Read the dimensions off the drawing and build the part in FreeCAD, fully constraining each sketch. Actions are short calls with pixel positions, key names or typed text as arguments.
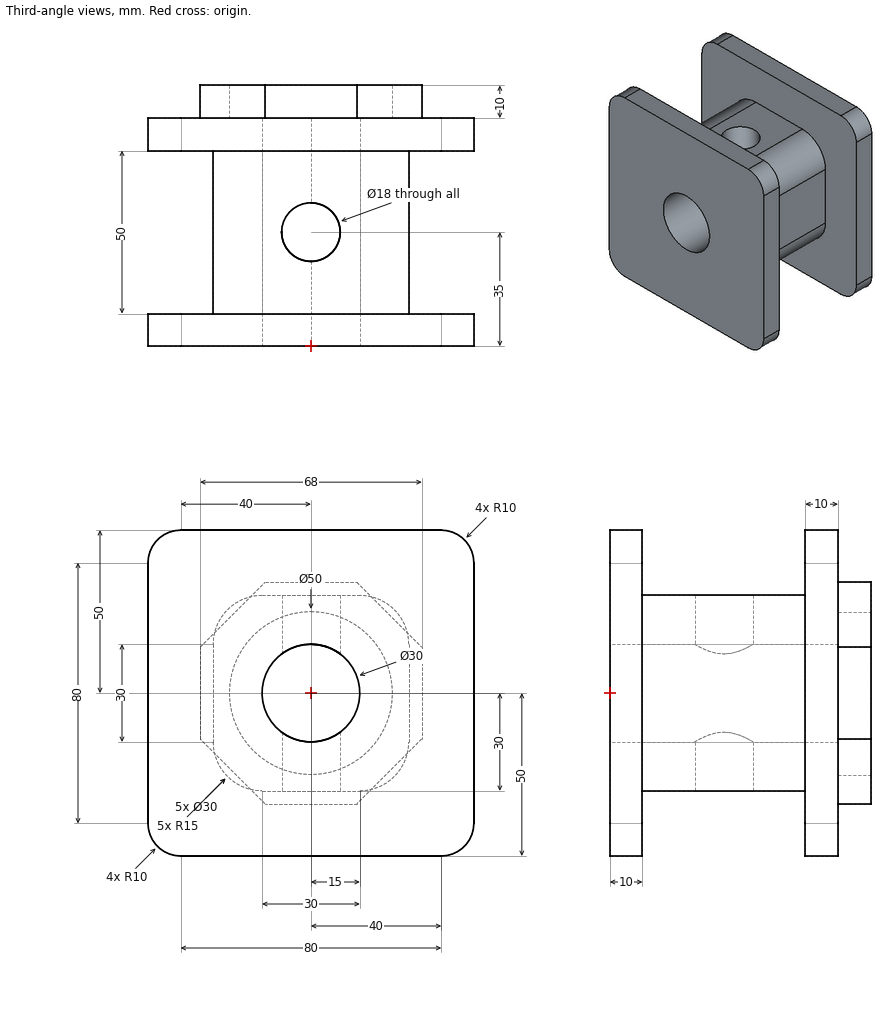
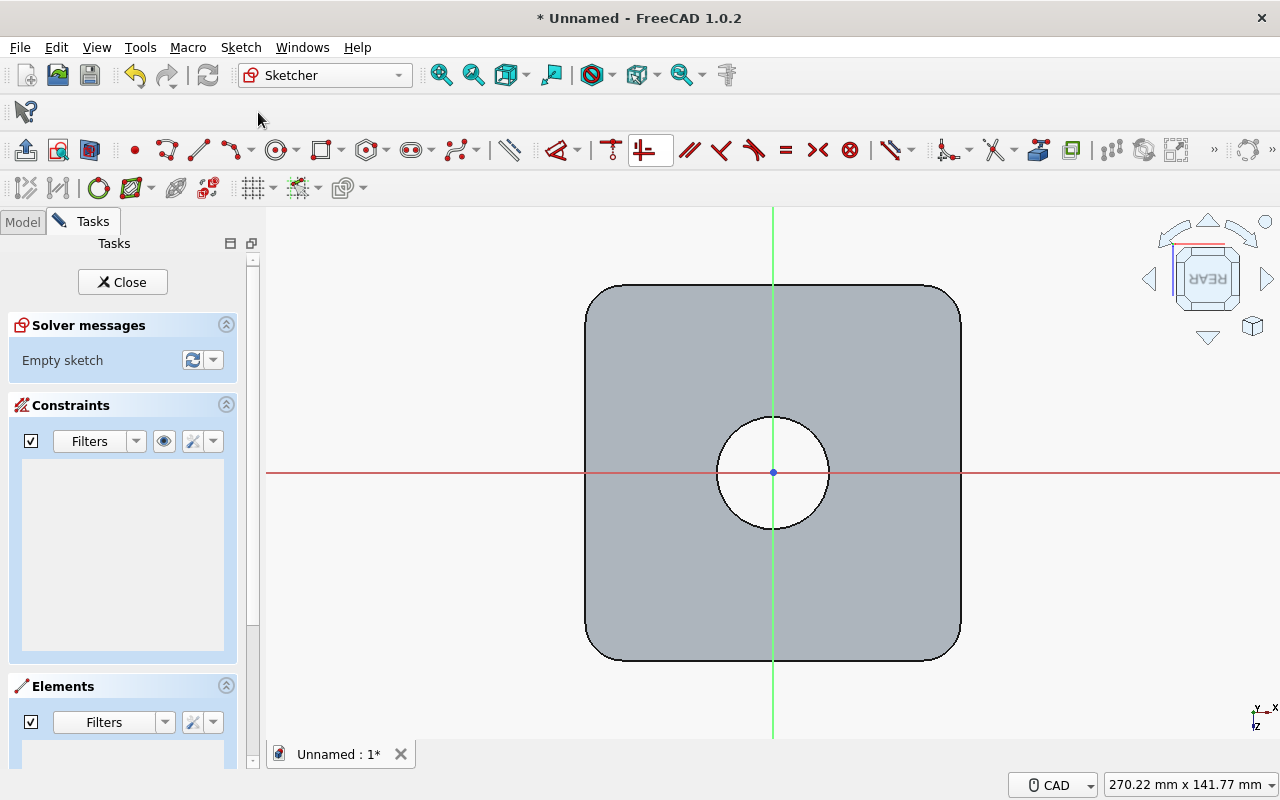
click(388, 150)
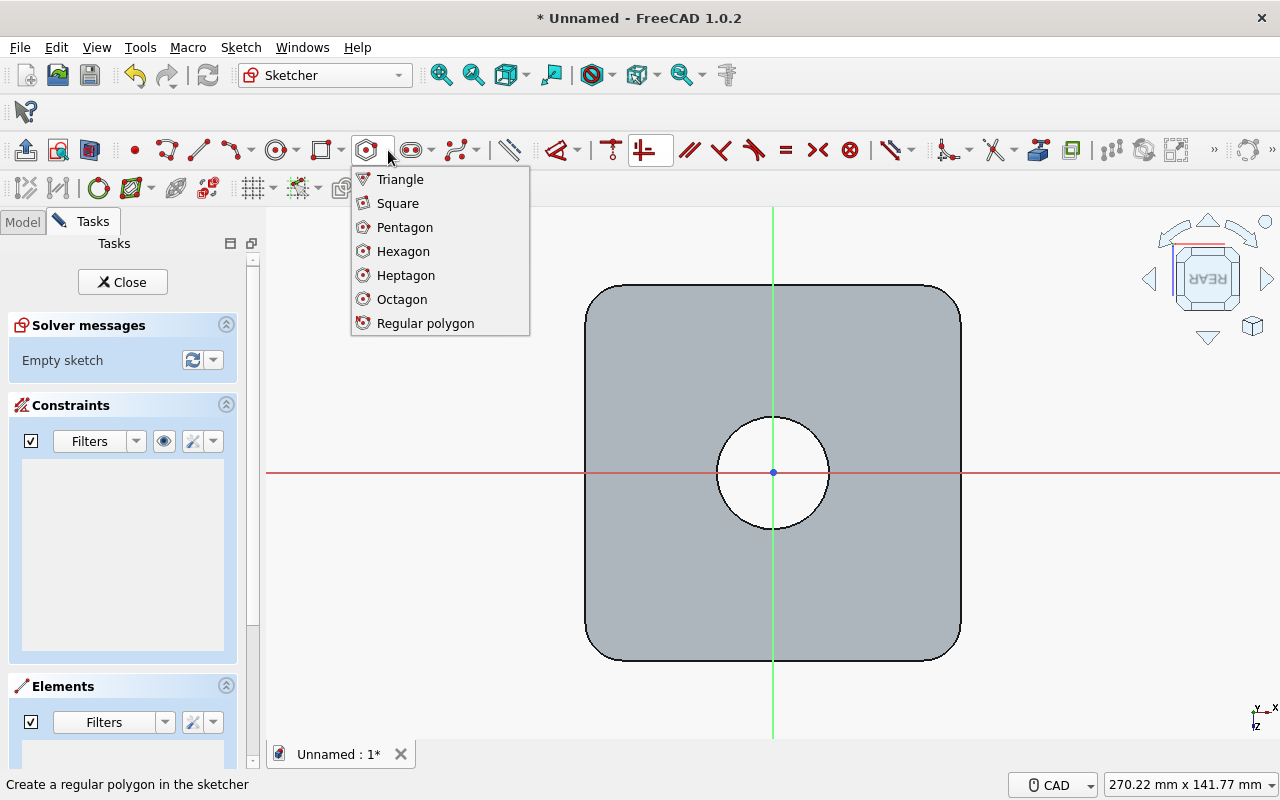
click(440, 299)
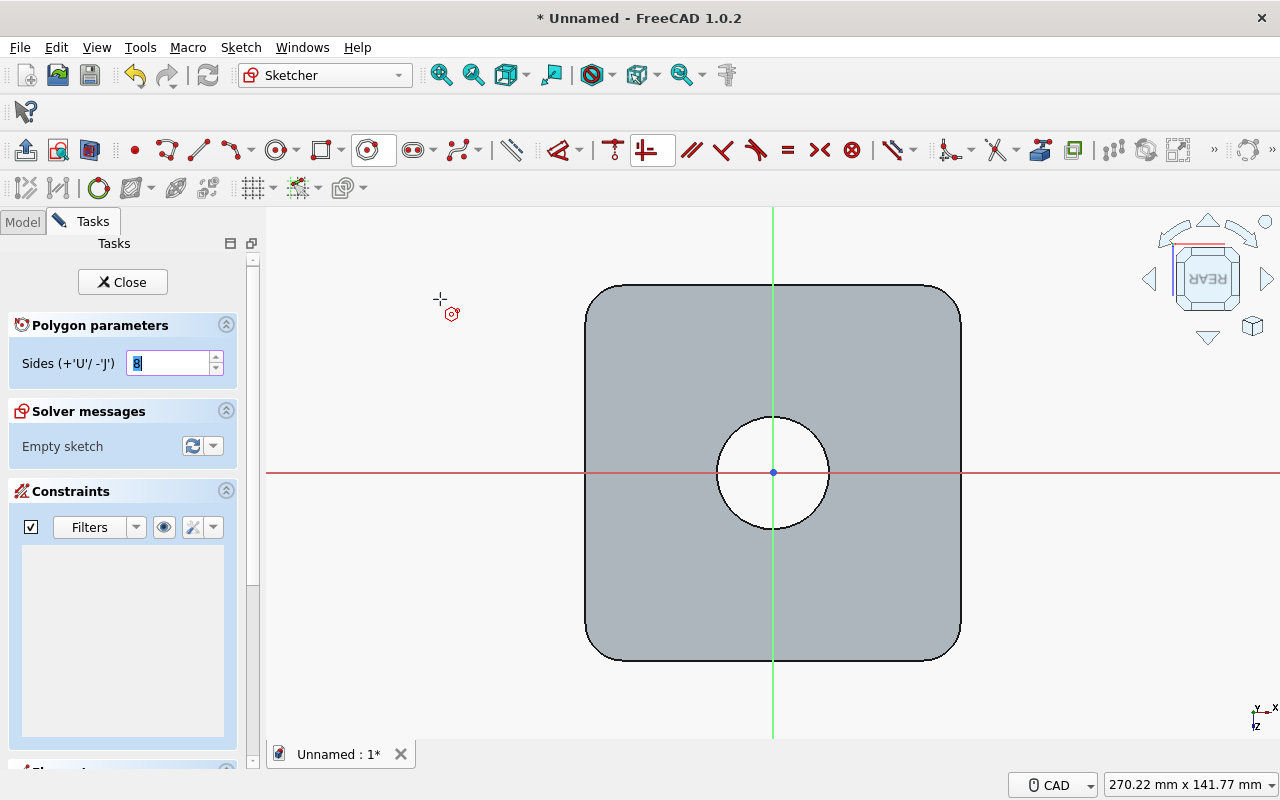
click(773, 473)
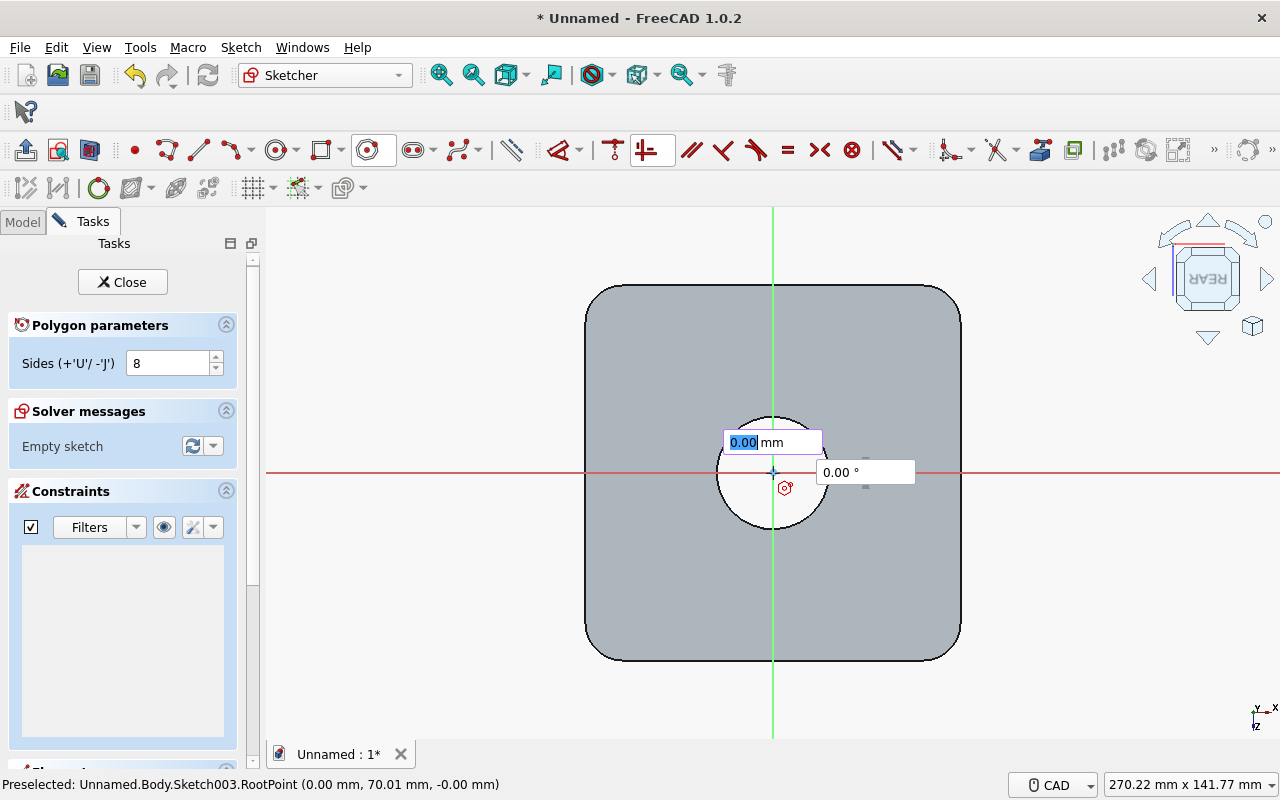
click(901, 526)
right_click(901, 526)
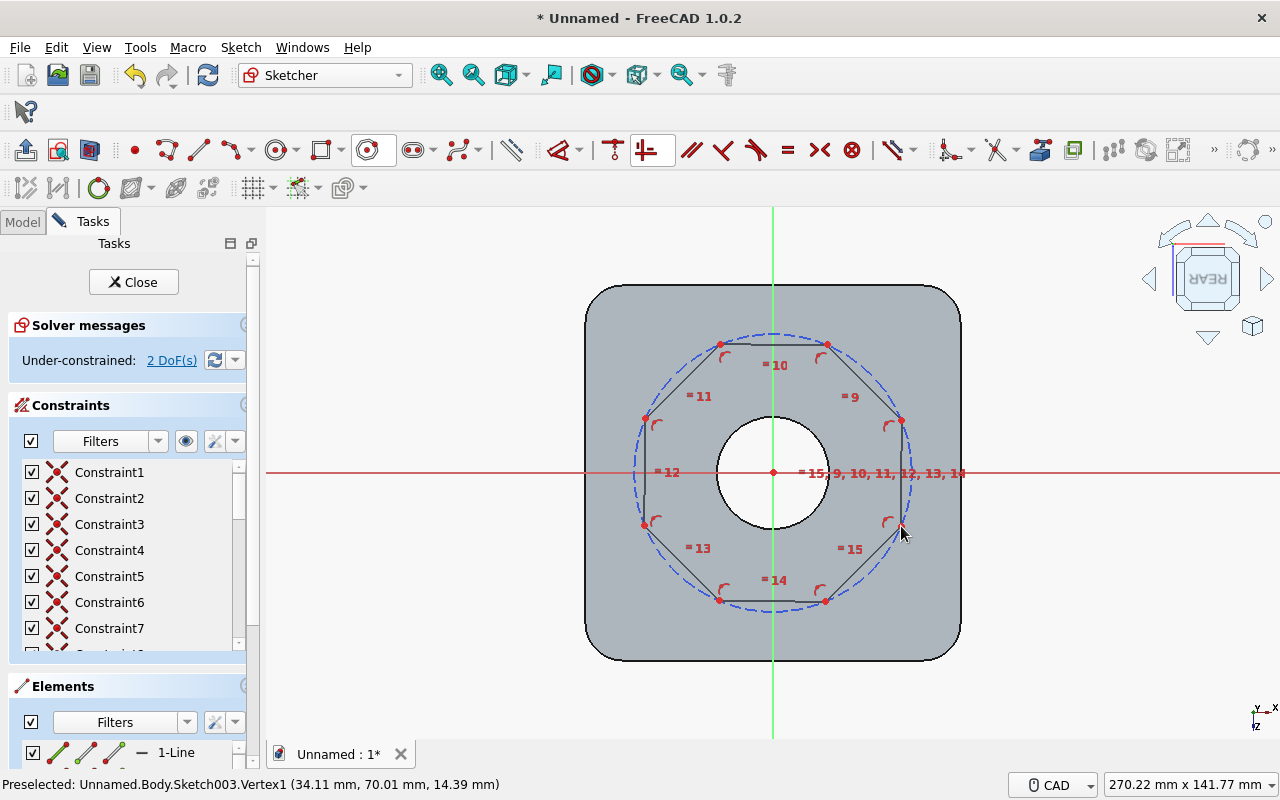
click(276, 150)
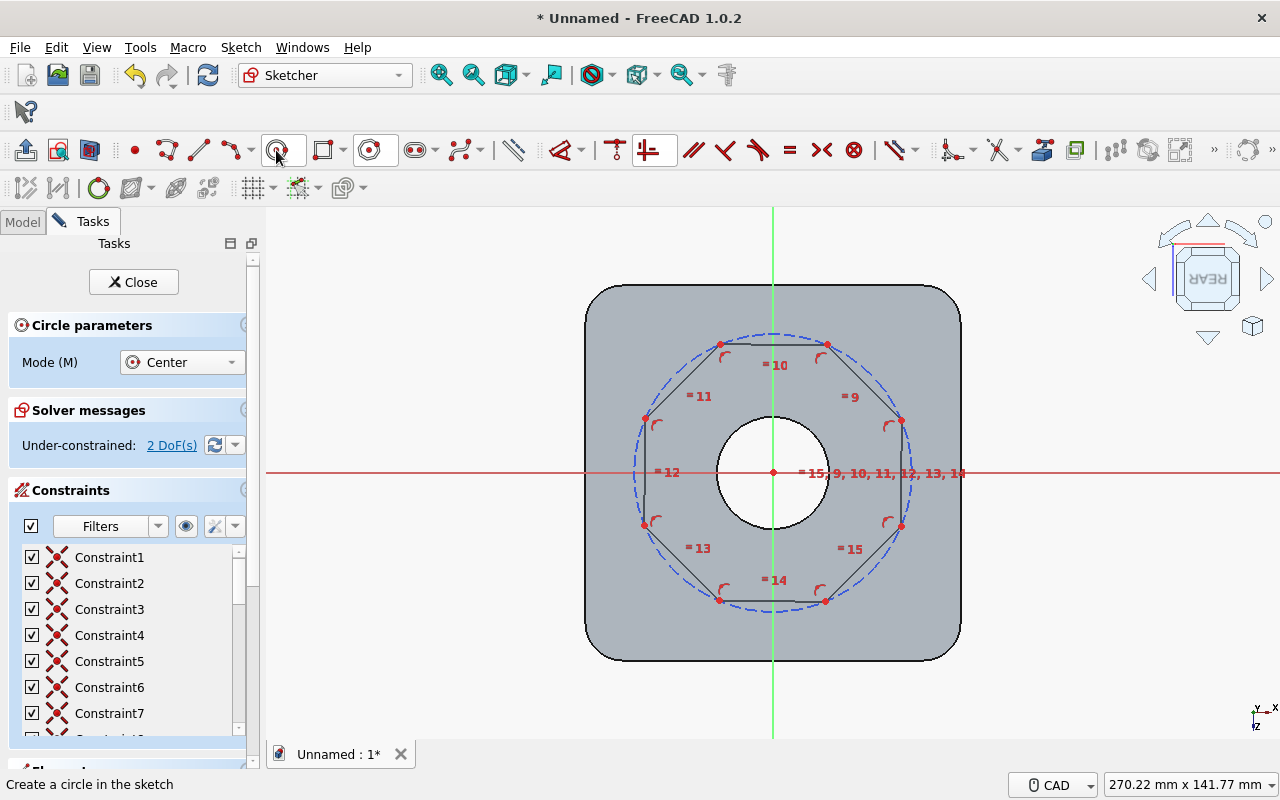
click(773, 473)
move(839, 407)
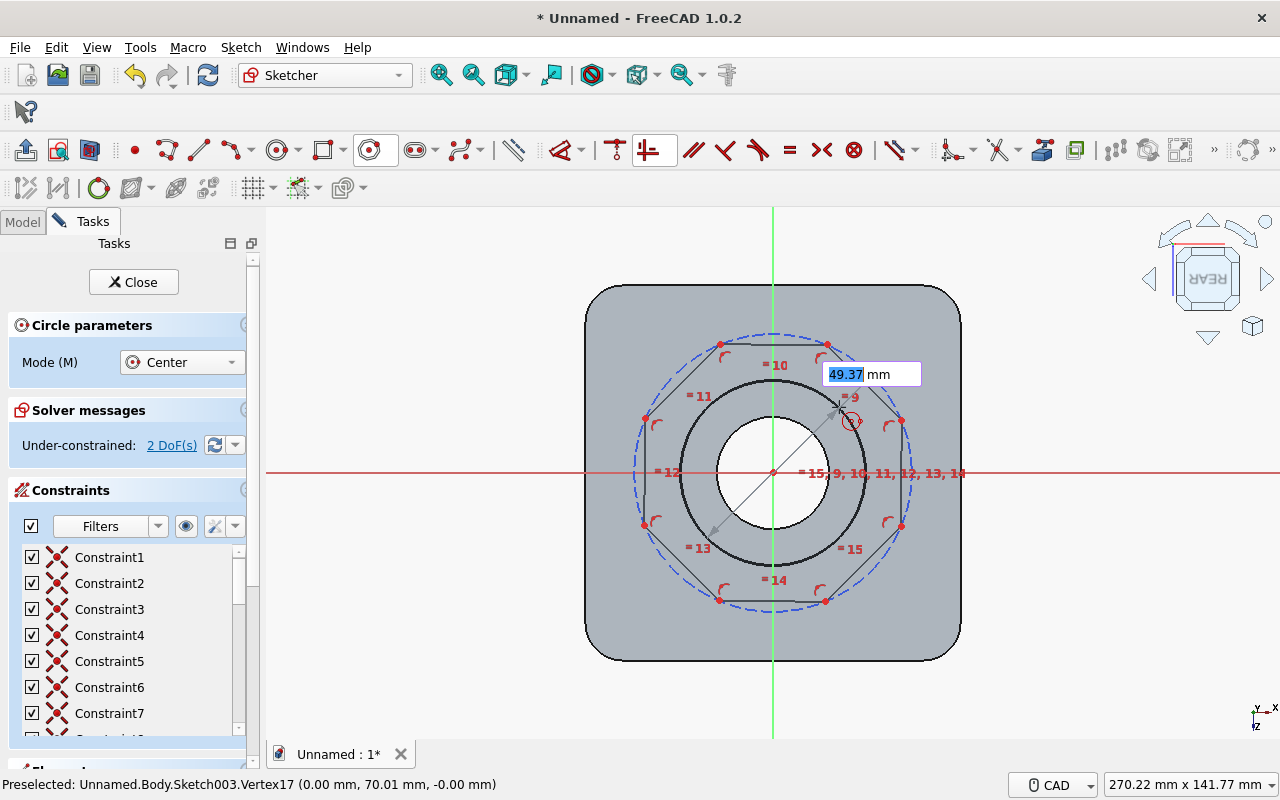
text(50)
key(Return)
key(Escape)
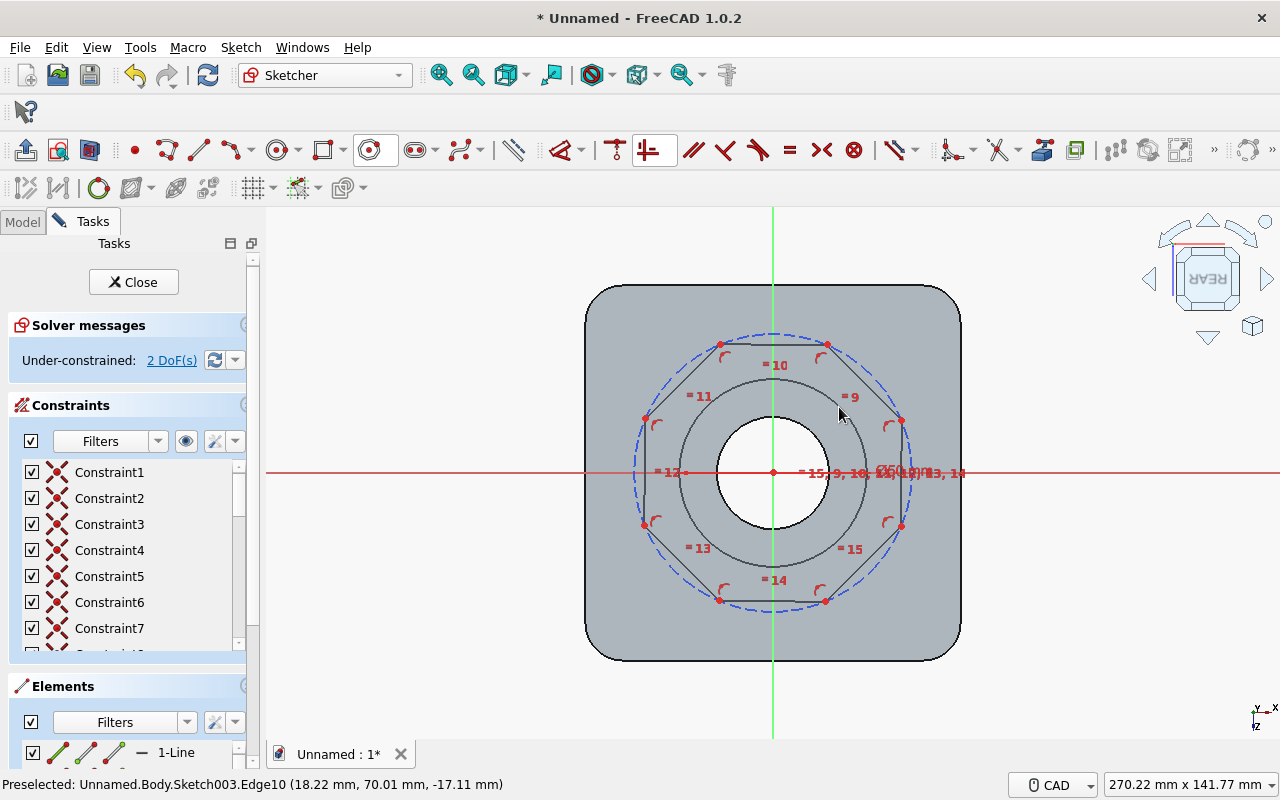
scroll(901, 484, up, 2)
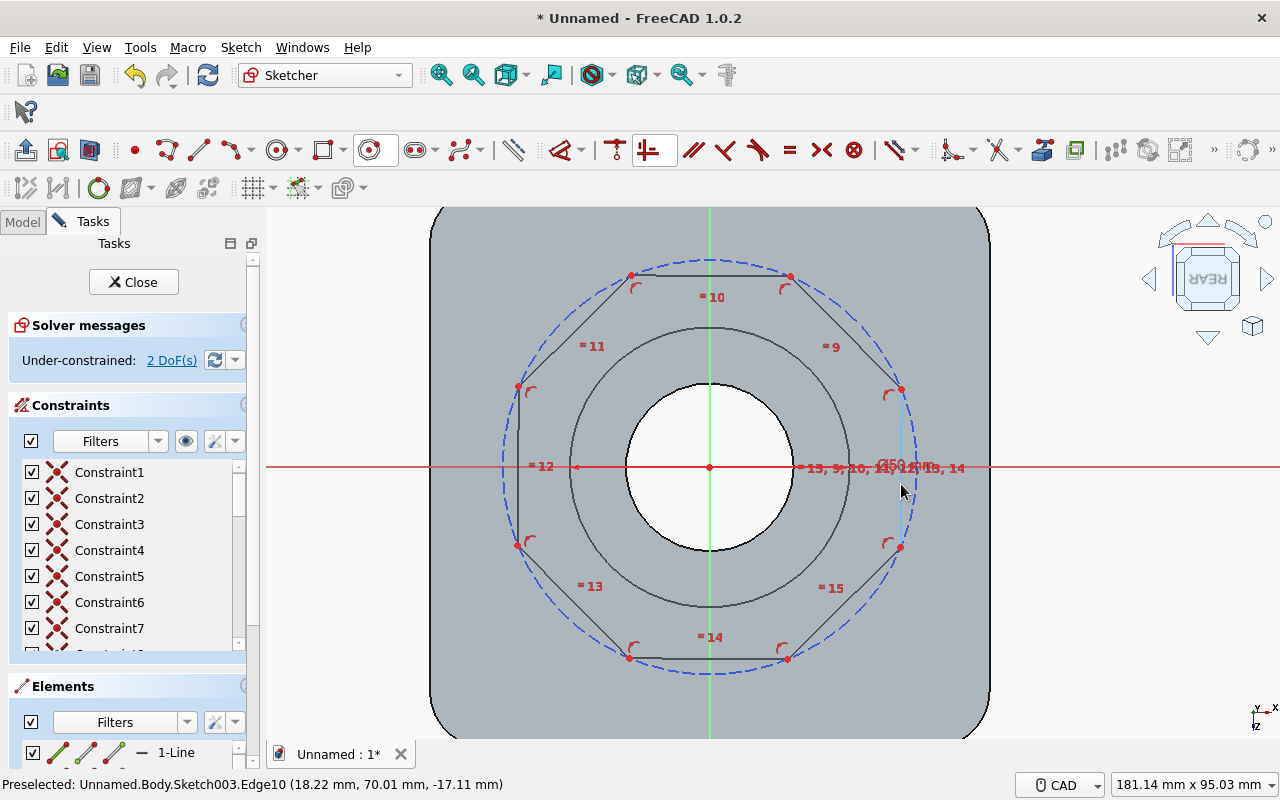
click(901, 484)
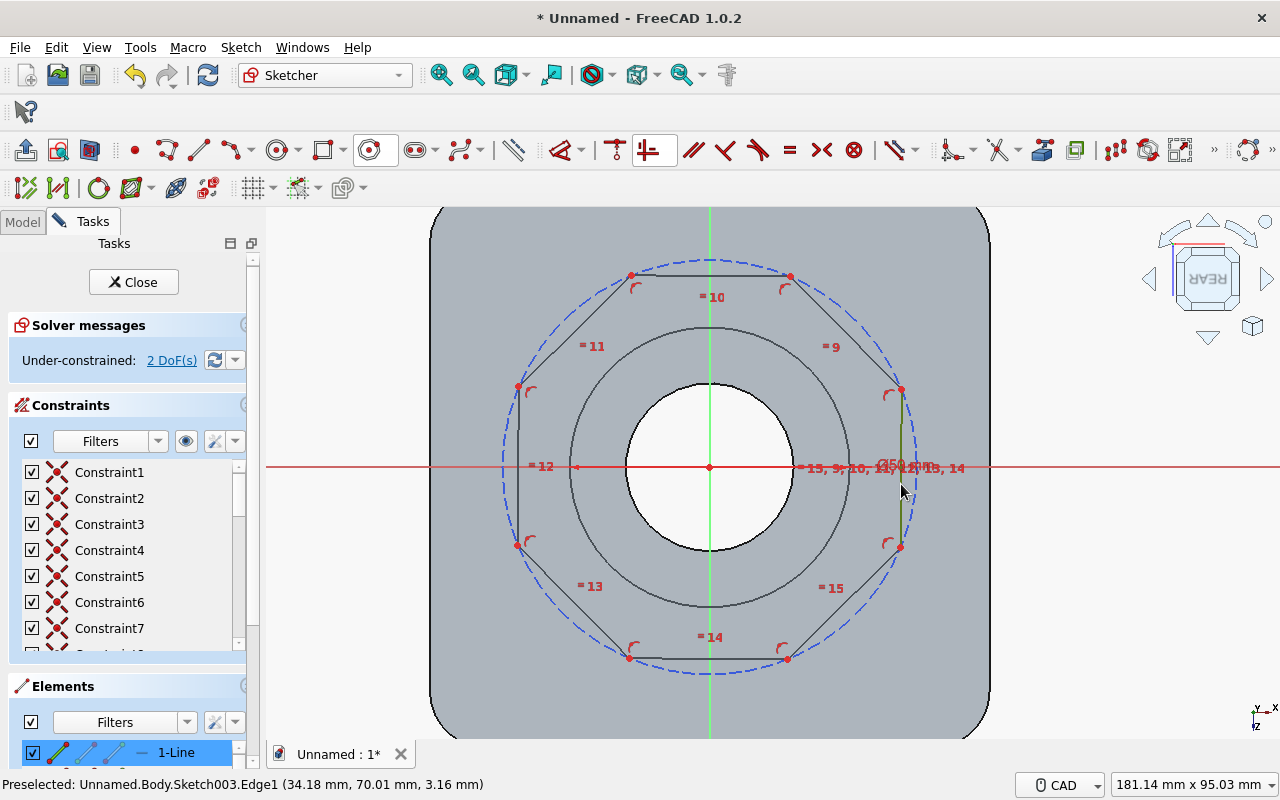
click(672, 150)